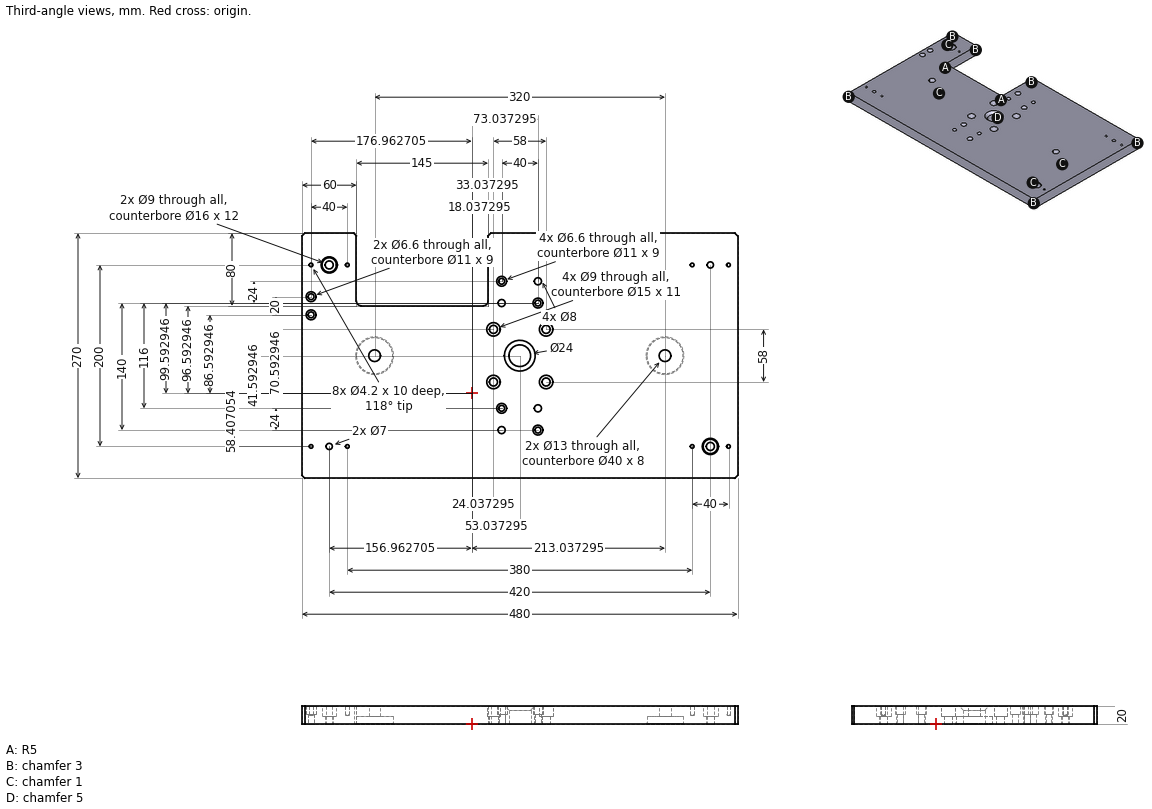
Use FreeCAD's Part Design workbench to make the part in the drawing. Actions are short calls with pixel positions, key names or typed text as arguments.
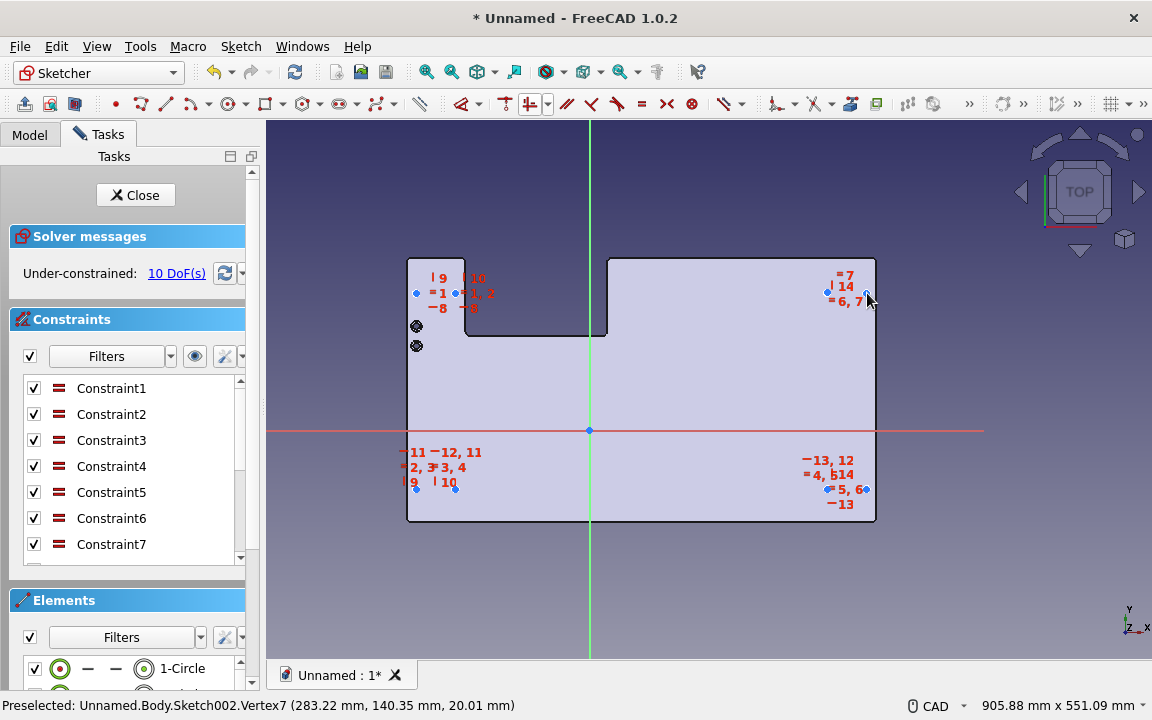
click(455, 294)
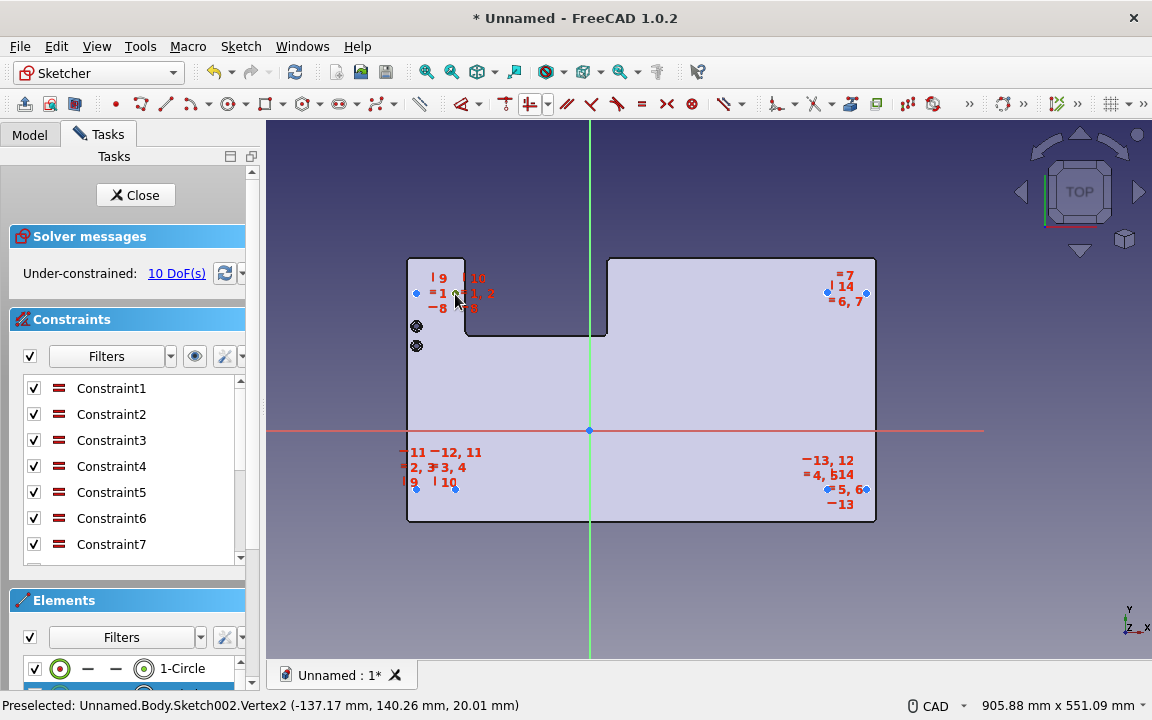
click(867, 293)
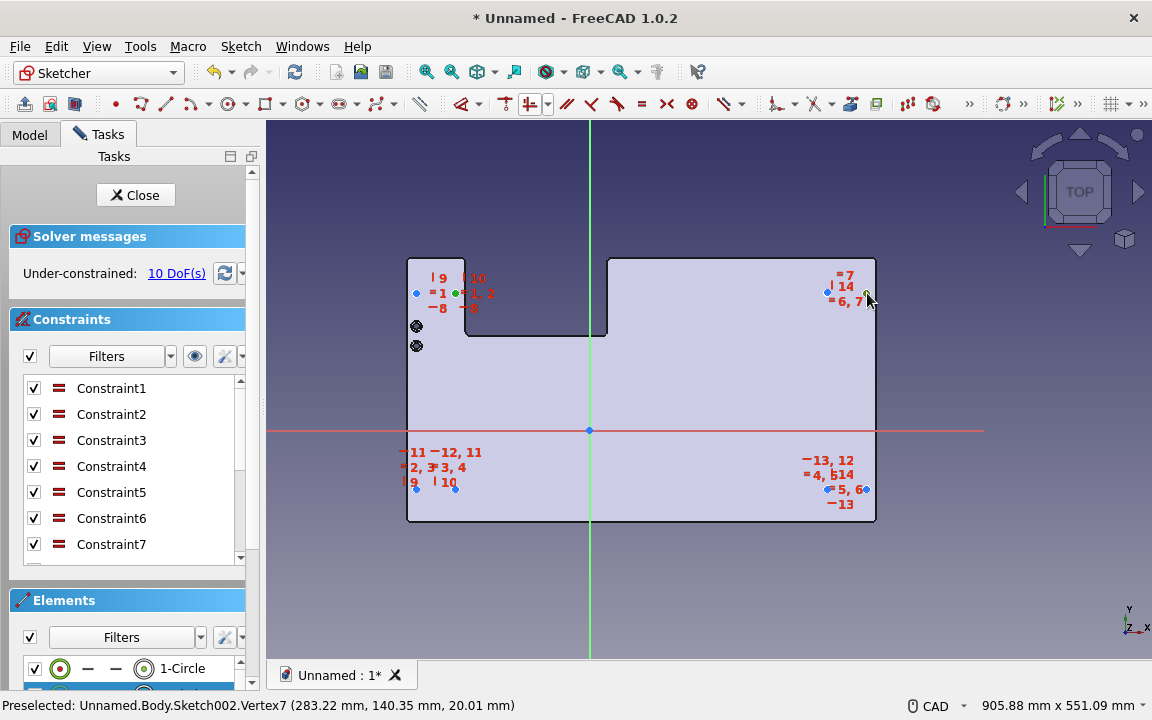
key(h)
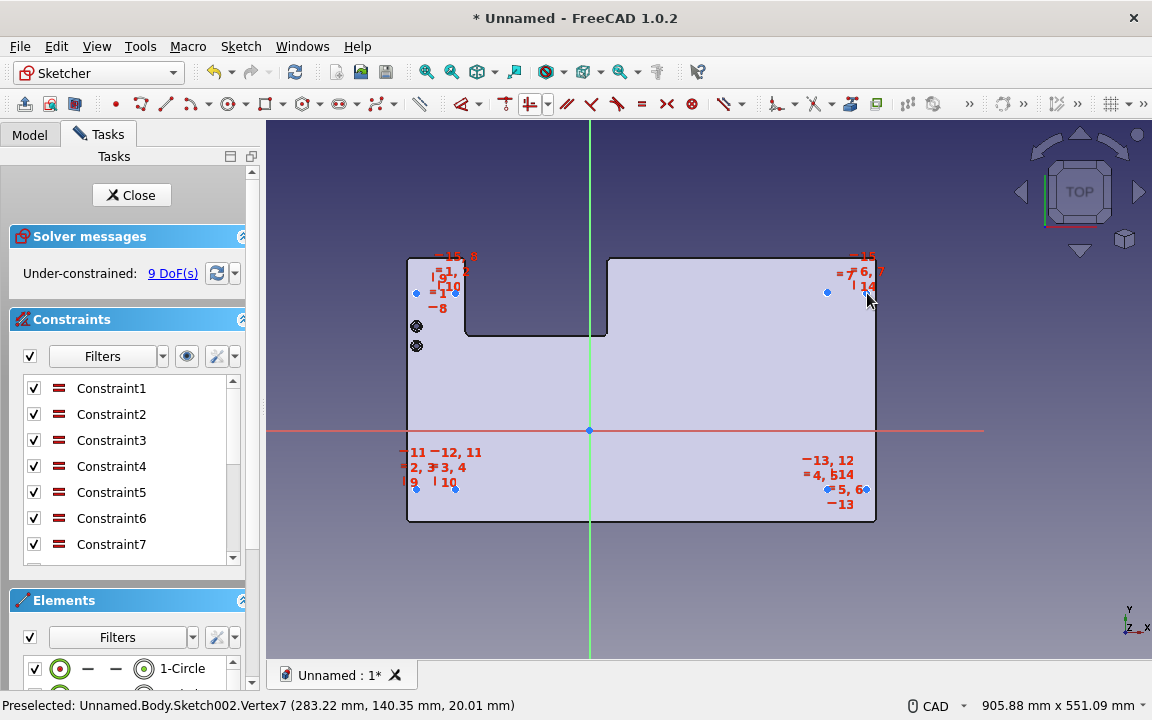
click(828, 489)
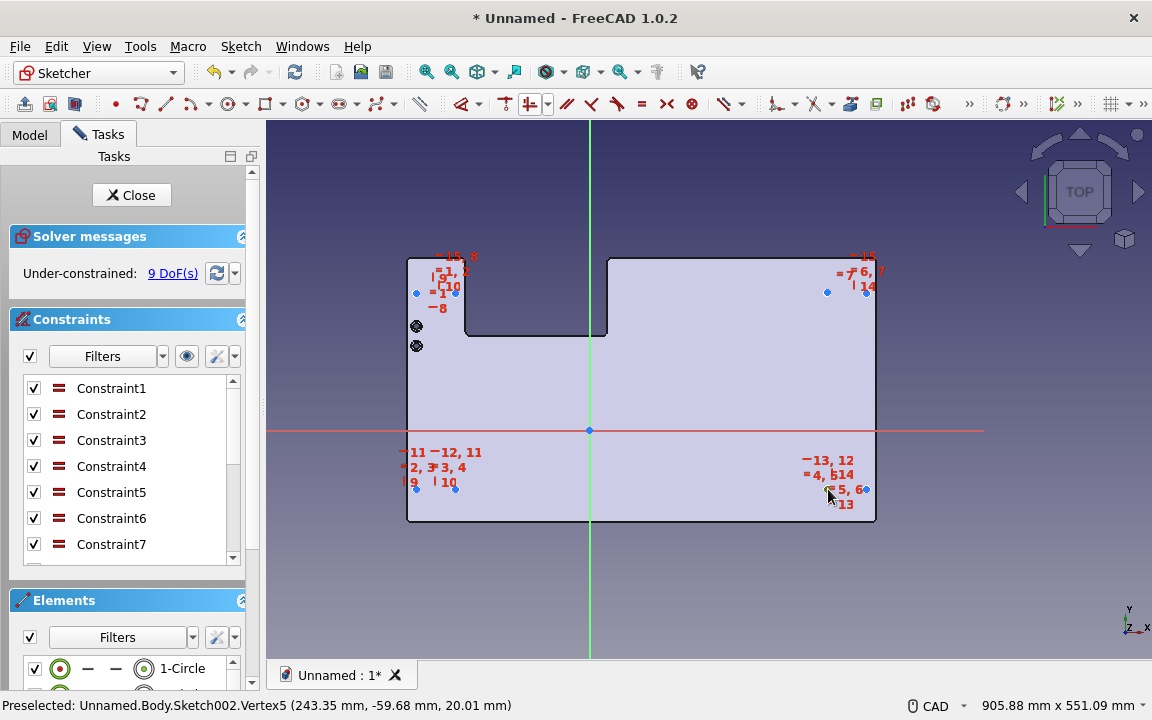
click(827, 293)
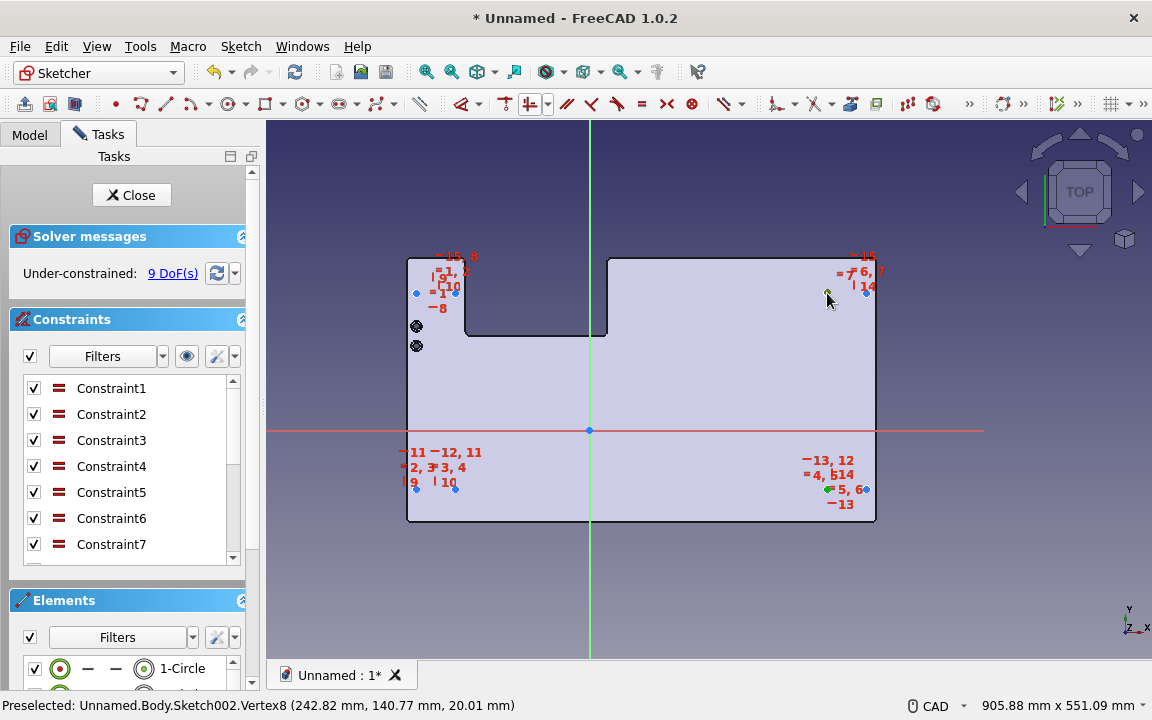
key(v)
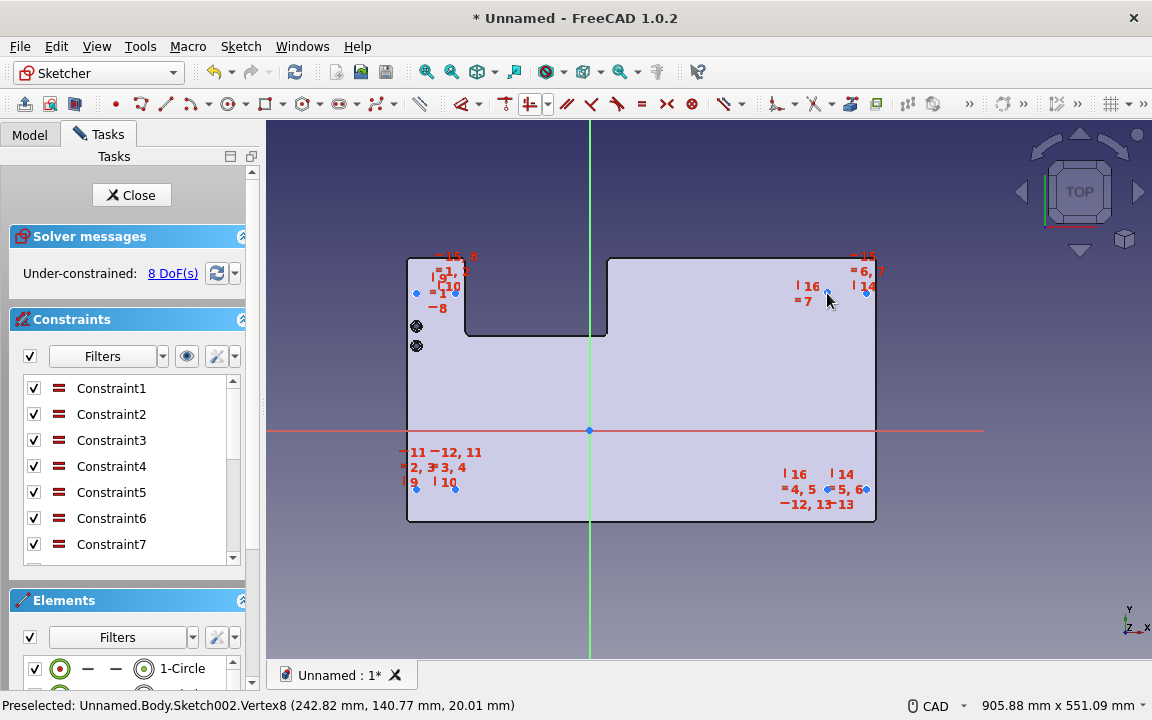
click(867, 294)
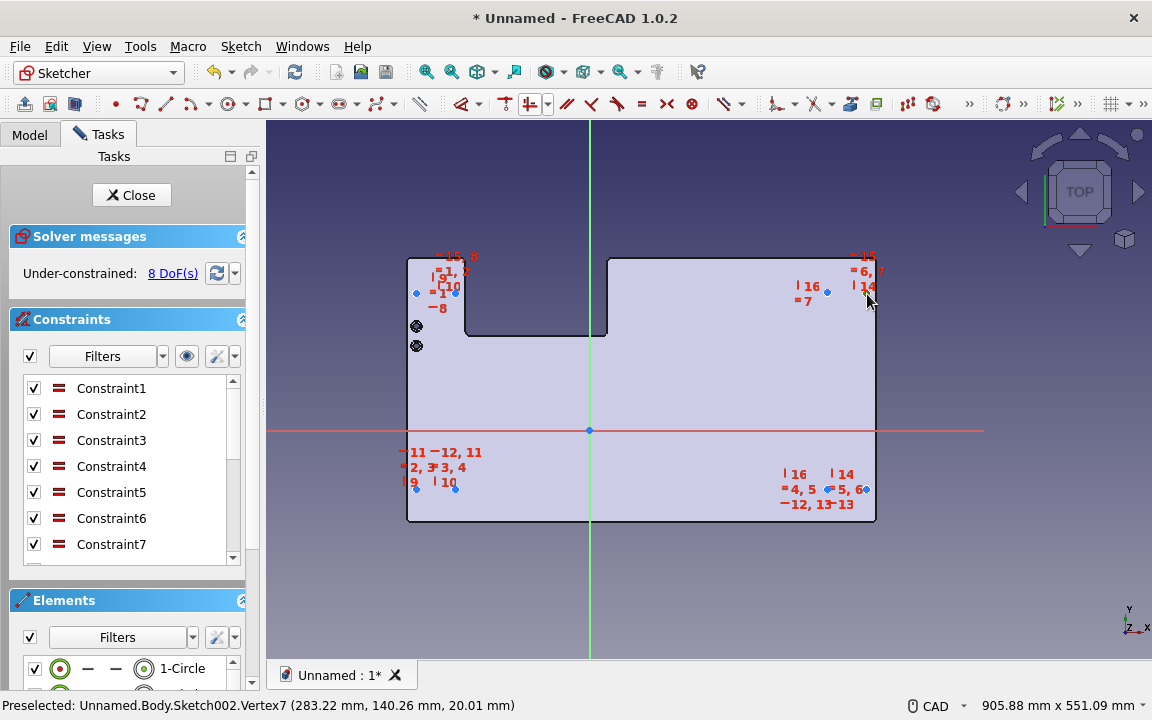
click(828, 293)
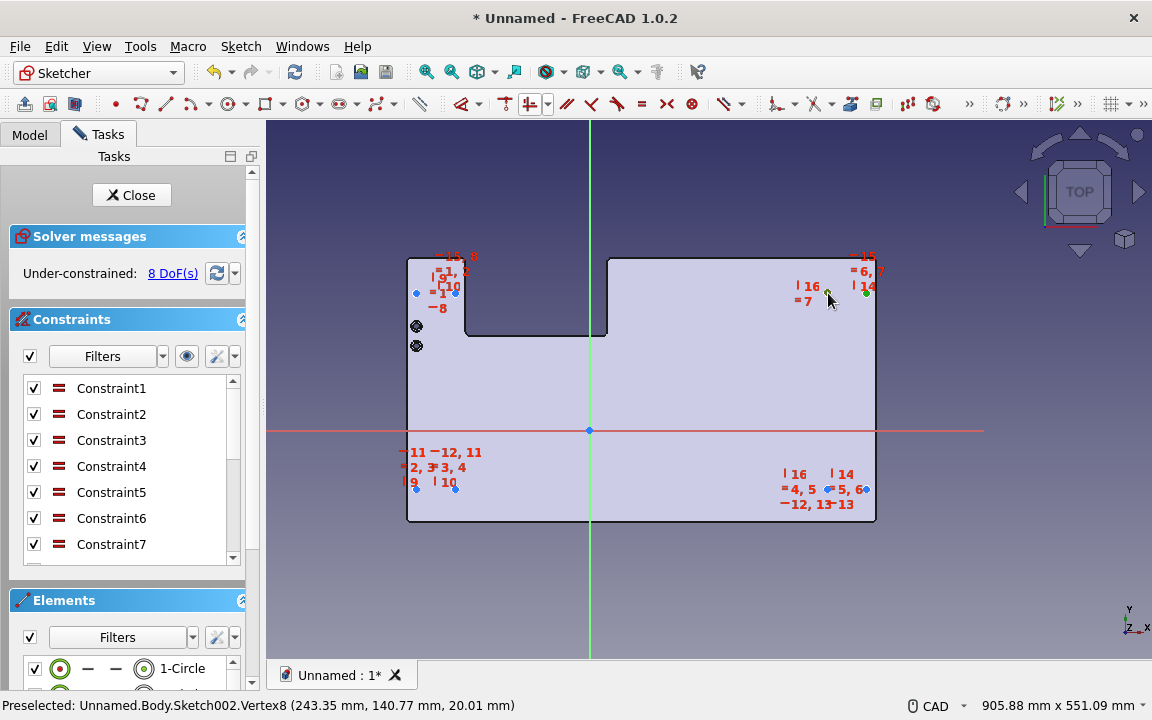
key(h)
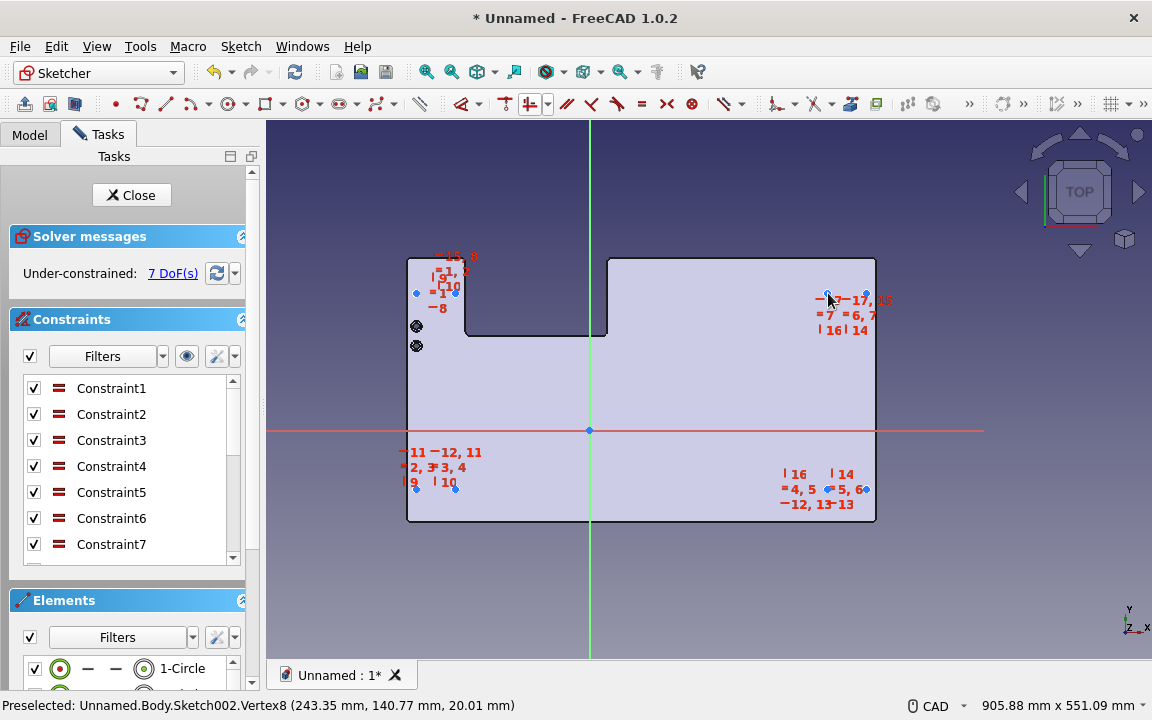
key(d)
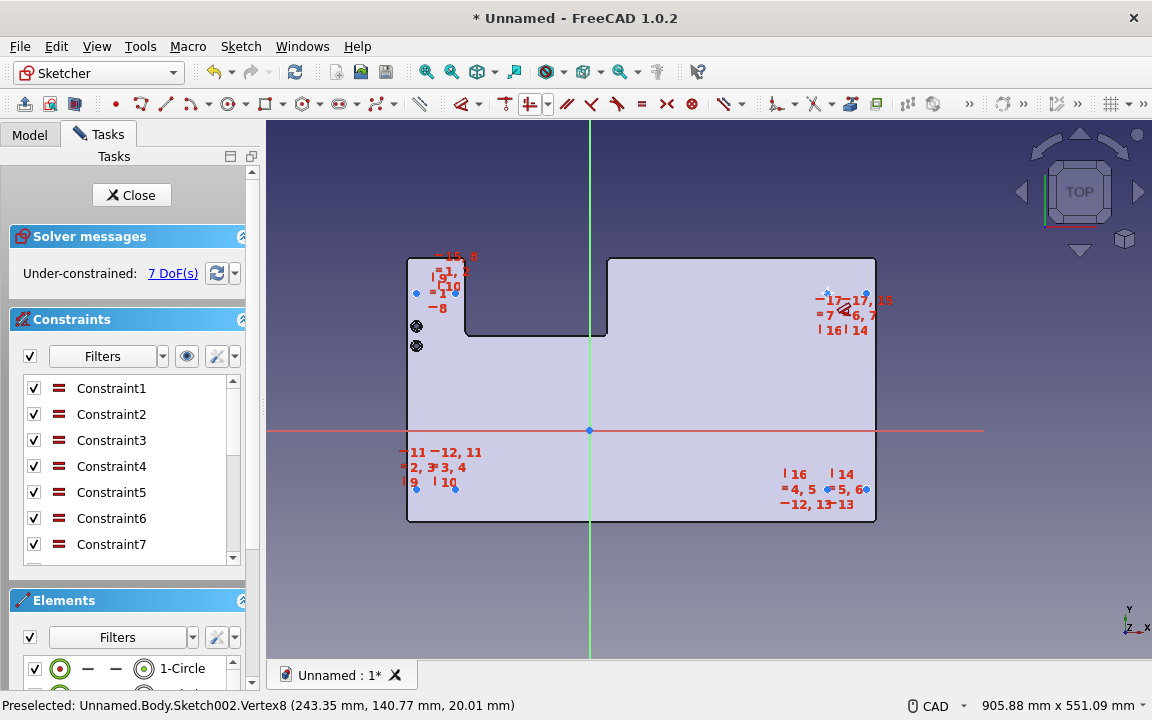
scroll(416, 290, up, 12)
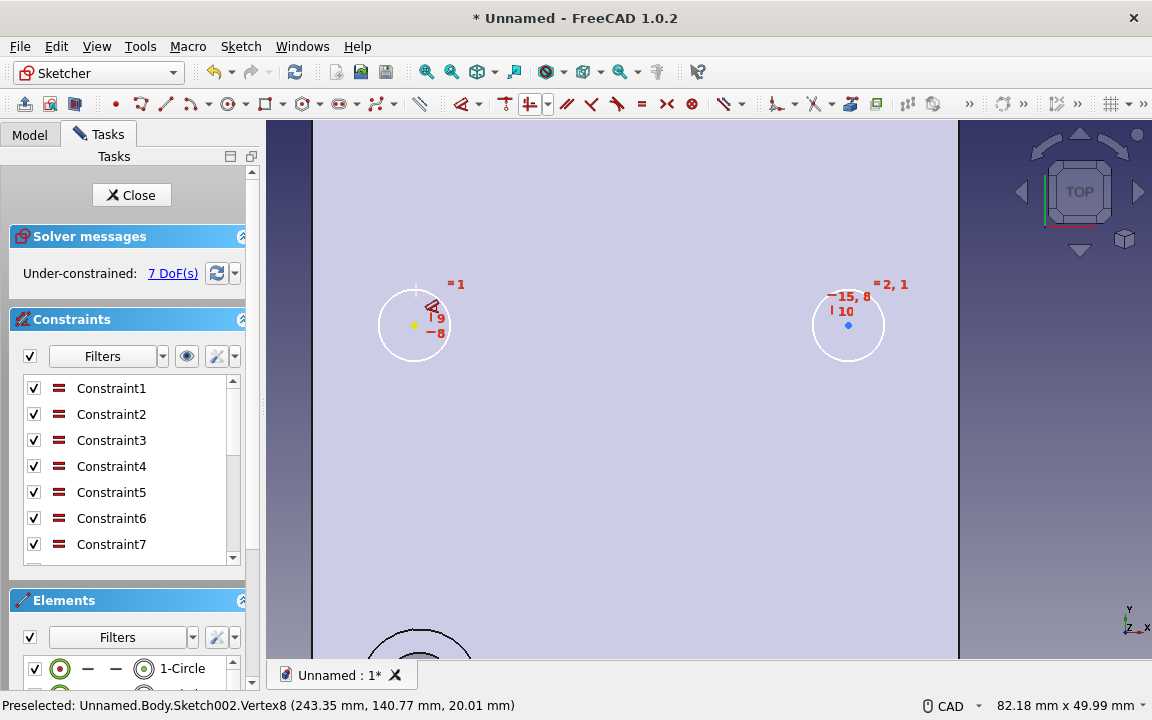
click(415, 290)
click(416, 258)